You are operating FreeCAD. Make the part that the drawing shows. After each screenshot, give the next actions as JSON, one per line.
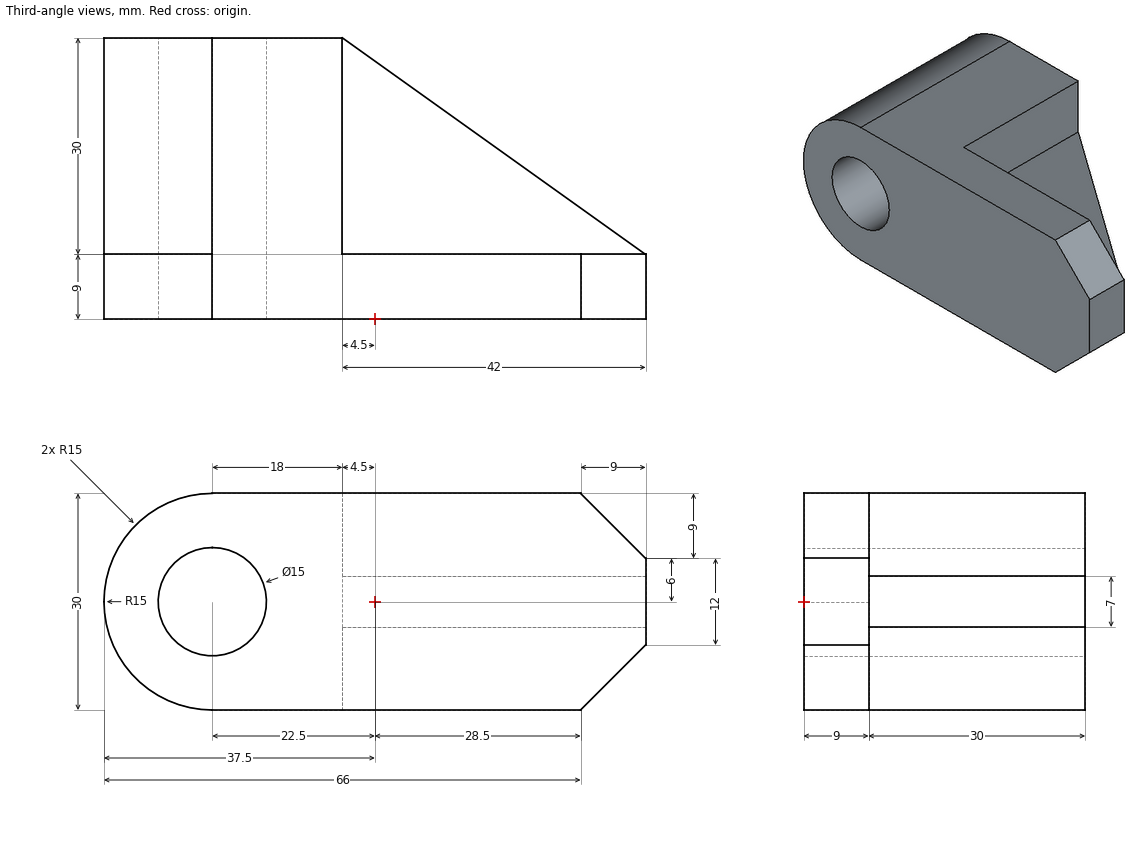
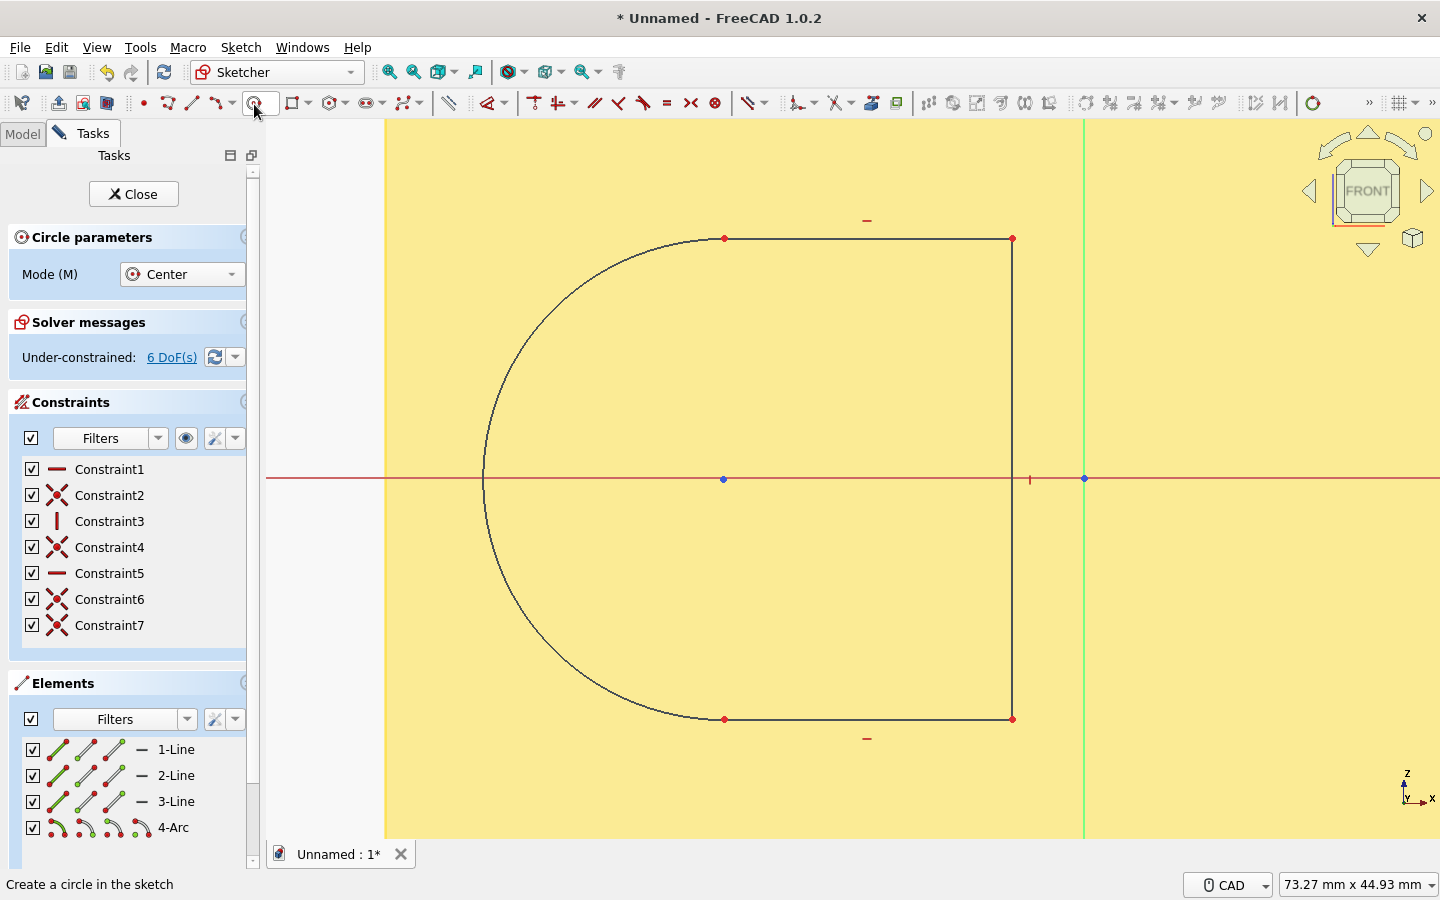
{"action": "left_click", "coordinate": [724, 478]}
{"action": "left_click", "coordinate": [809, 393]}
{"action": "key", "text": "Escape"}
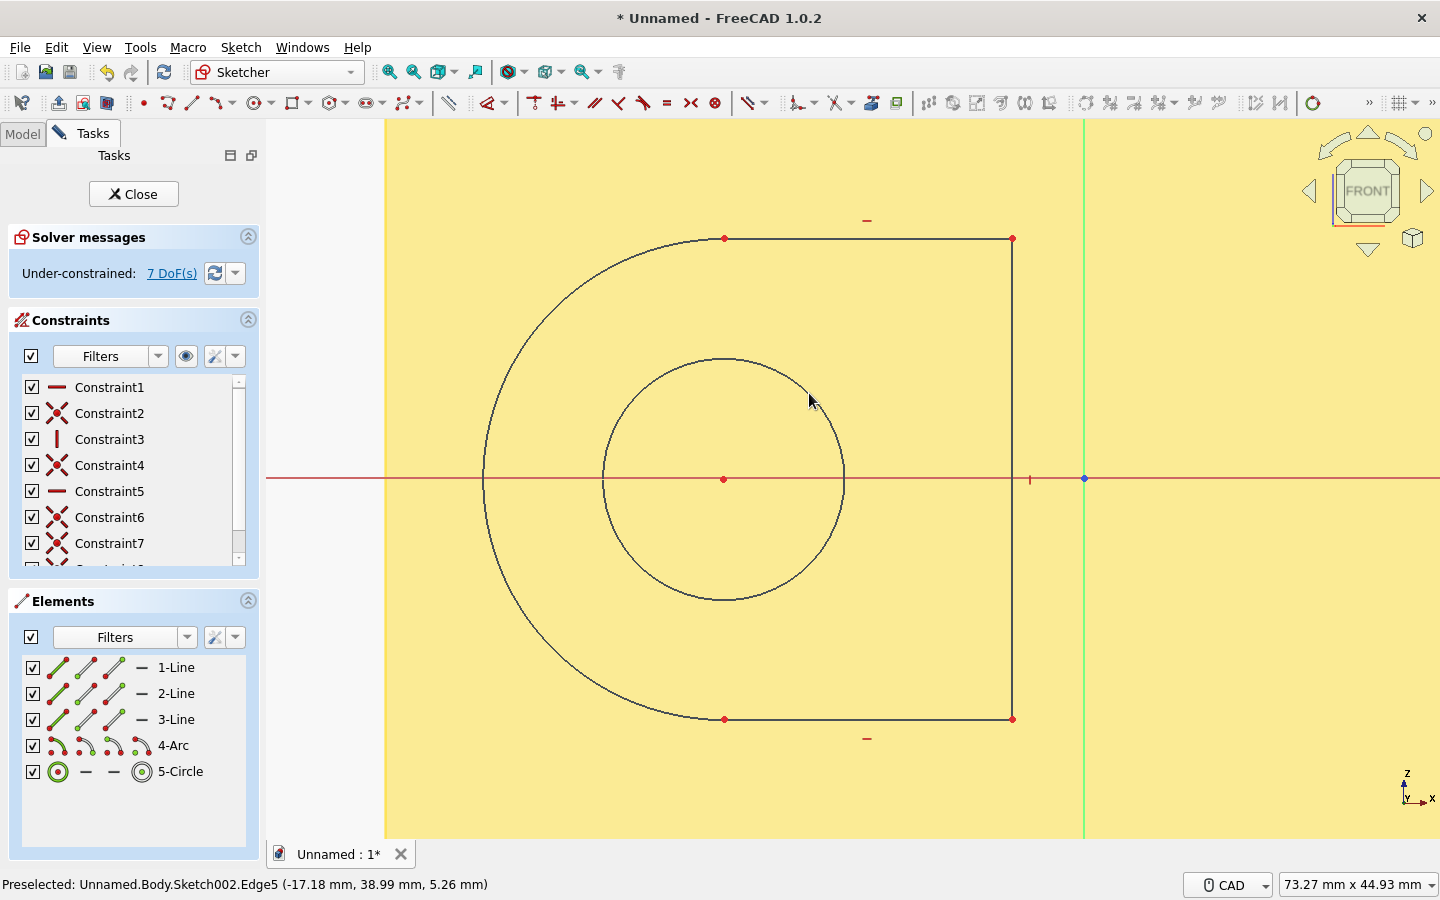
{"action": "left_click", "coordinate": [810, 239]}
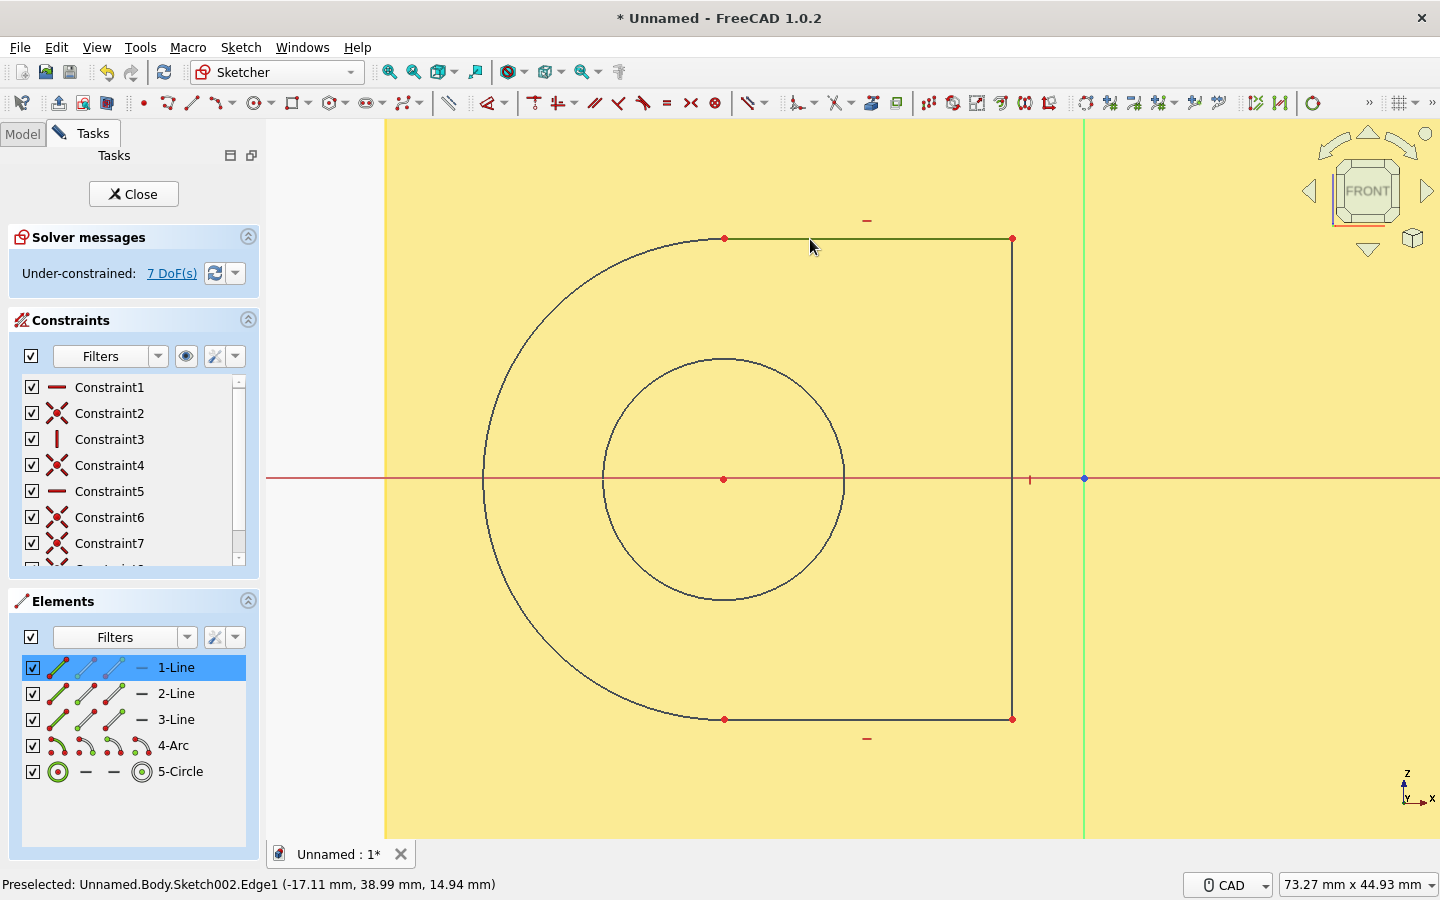
{"action": "left_click", "coordinate": [529, 338]}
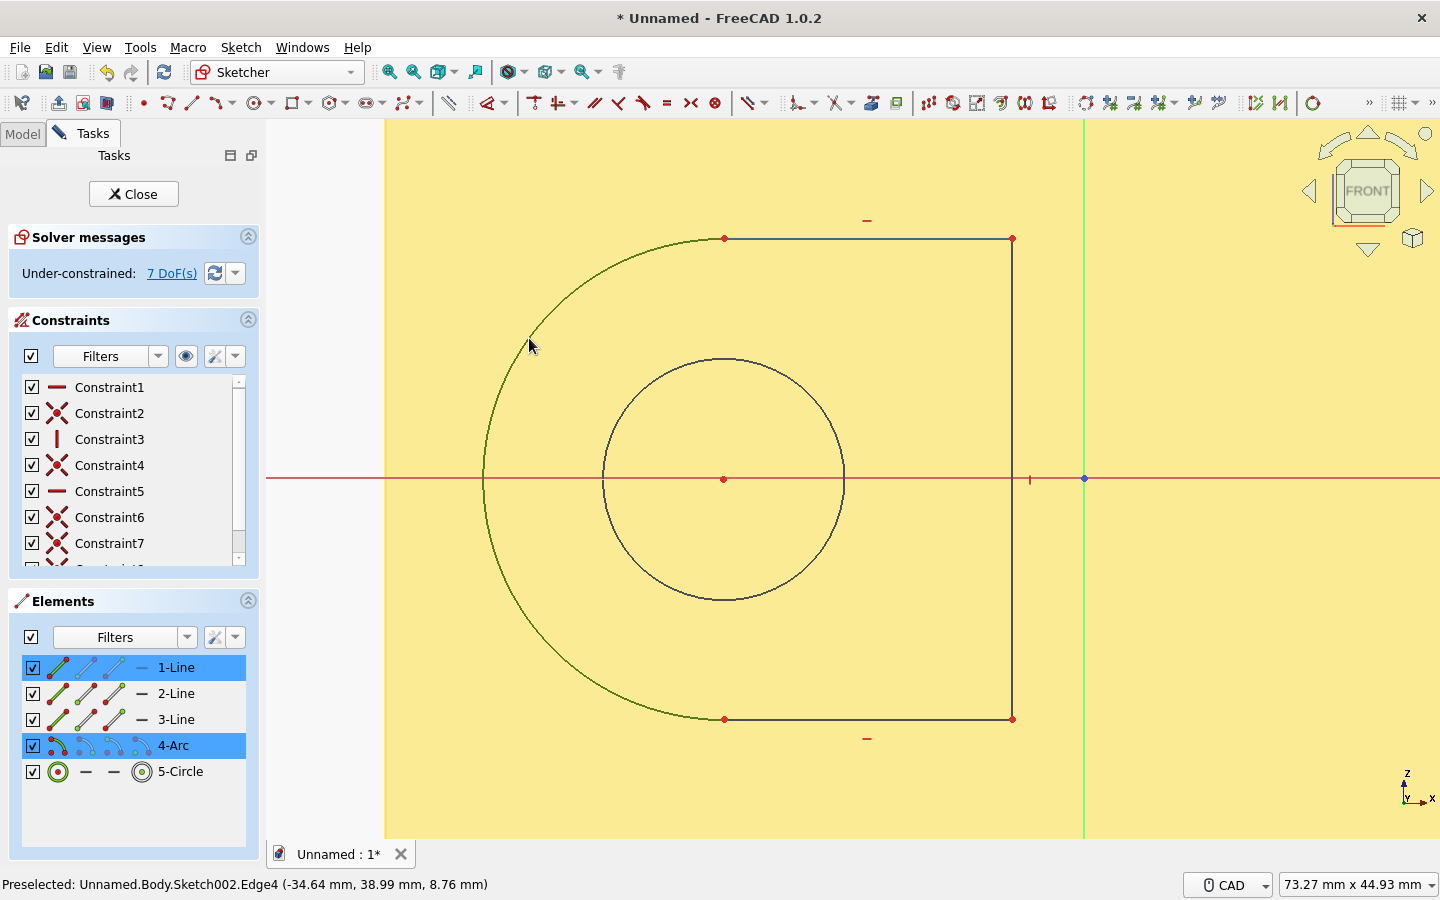
{"action": "left_click", "coordinate": [644, 104]}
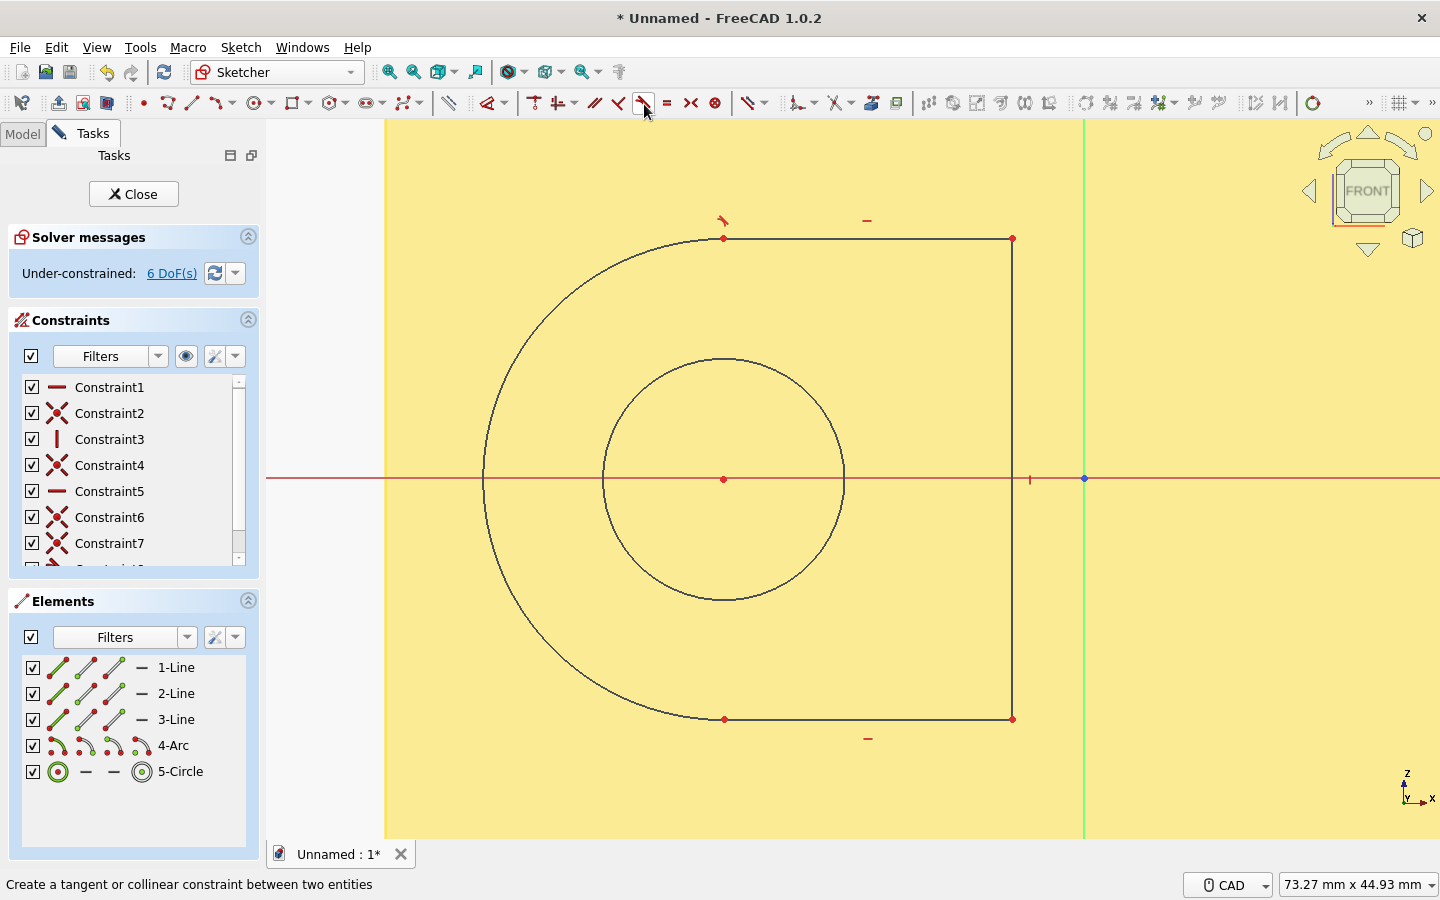
{"action": "left_click", "coordinate": [926, 720]}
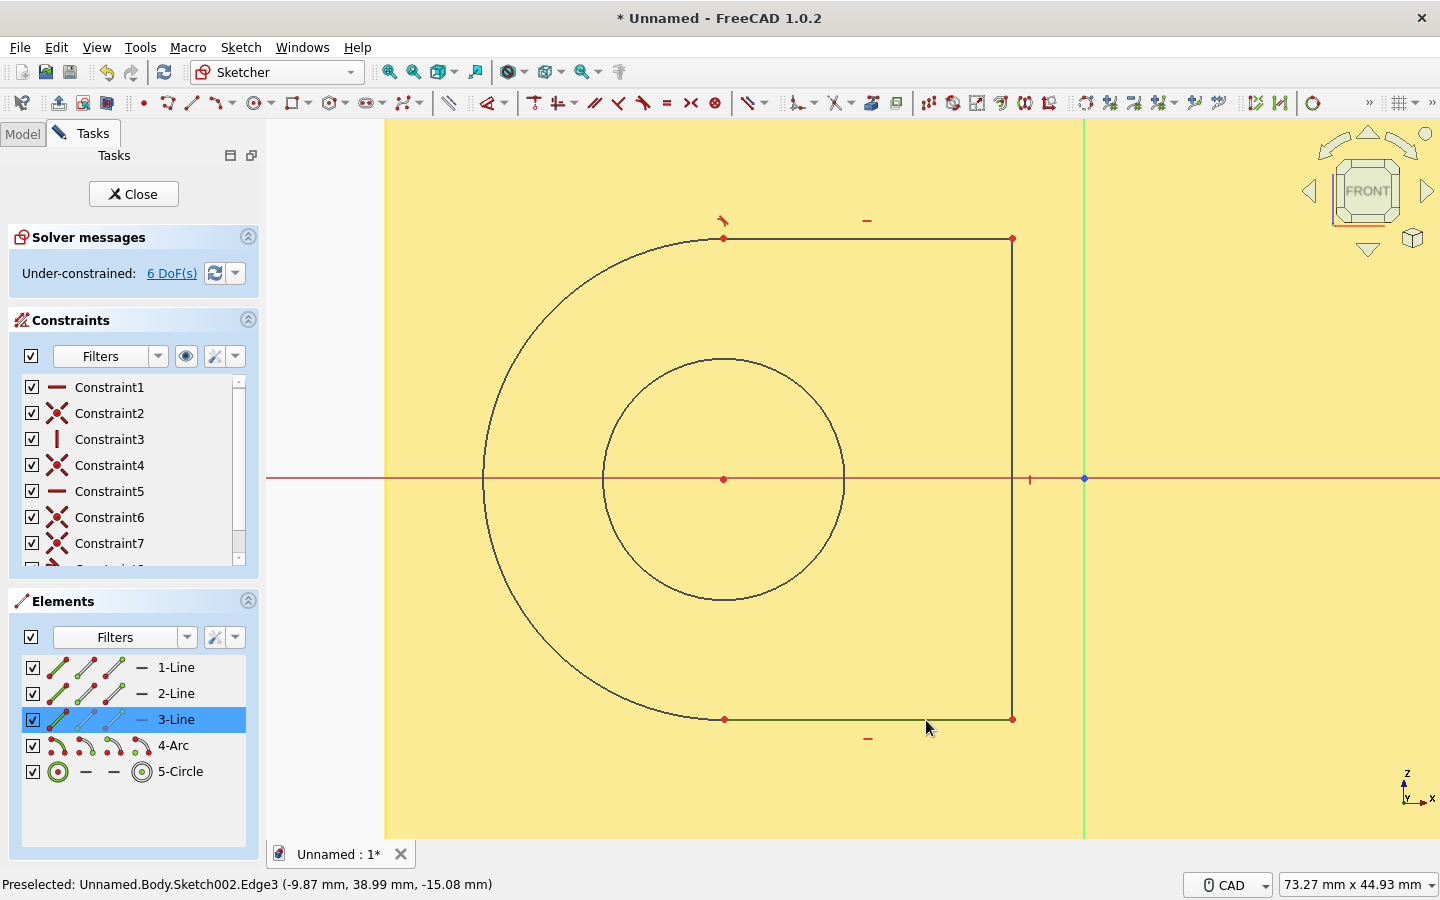
{"action": "left_click", "coordinate": [529, 338]}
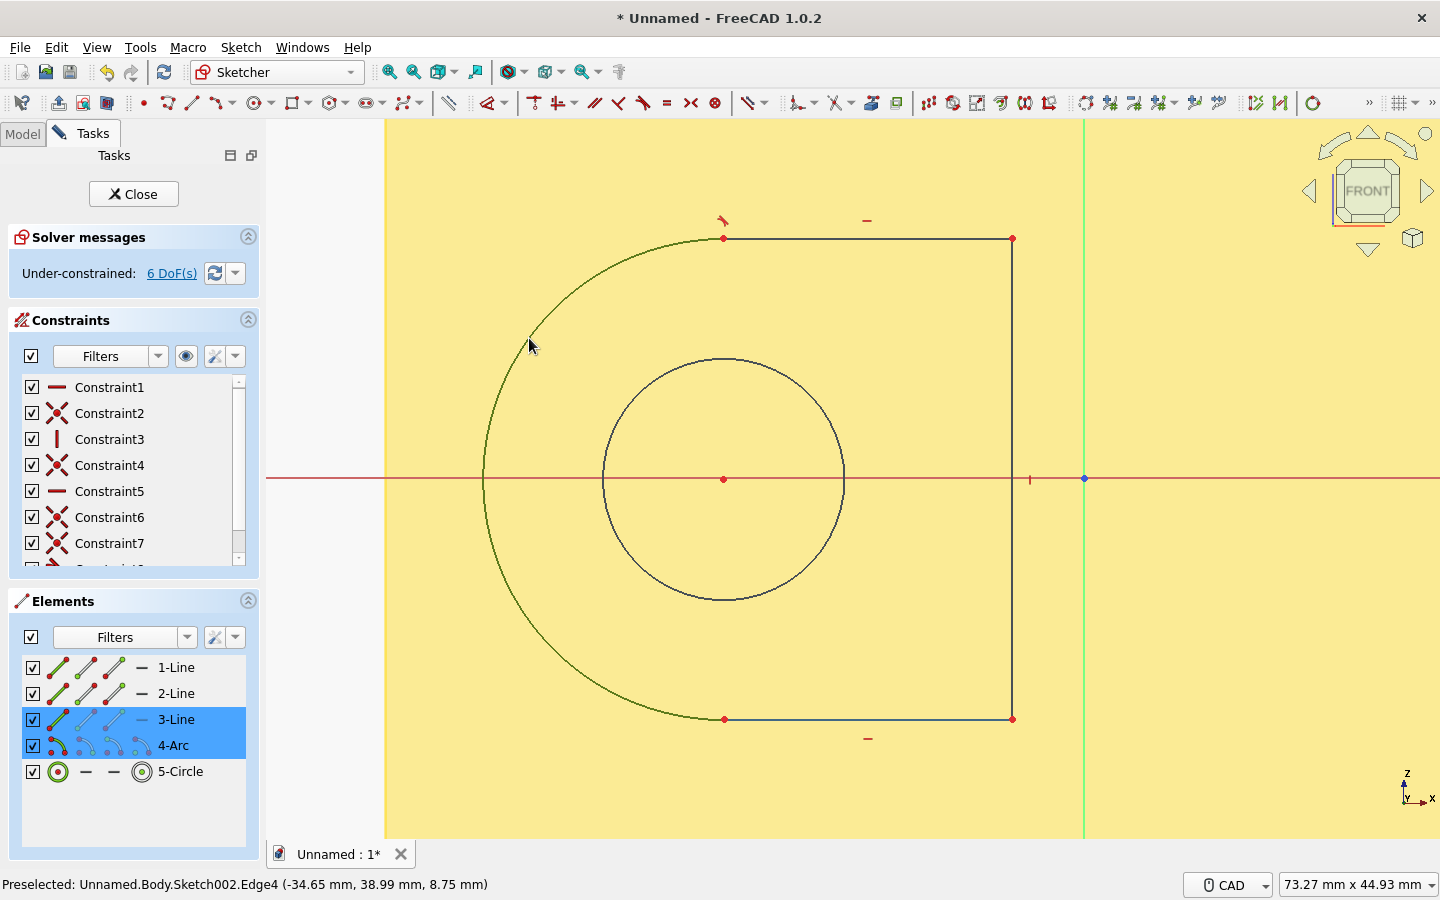
{"action": "key", "text": "t"}